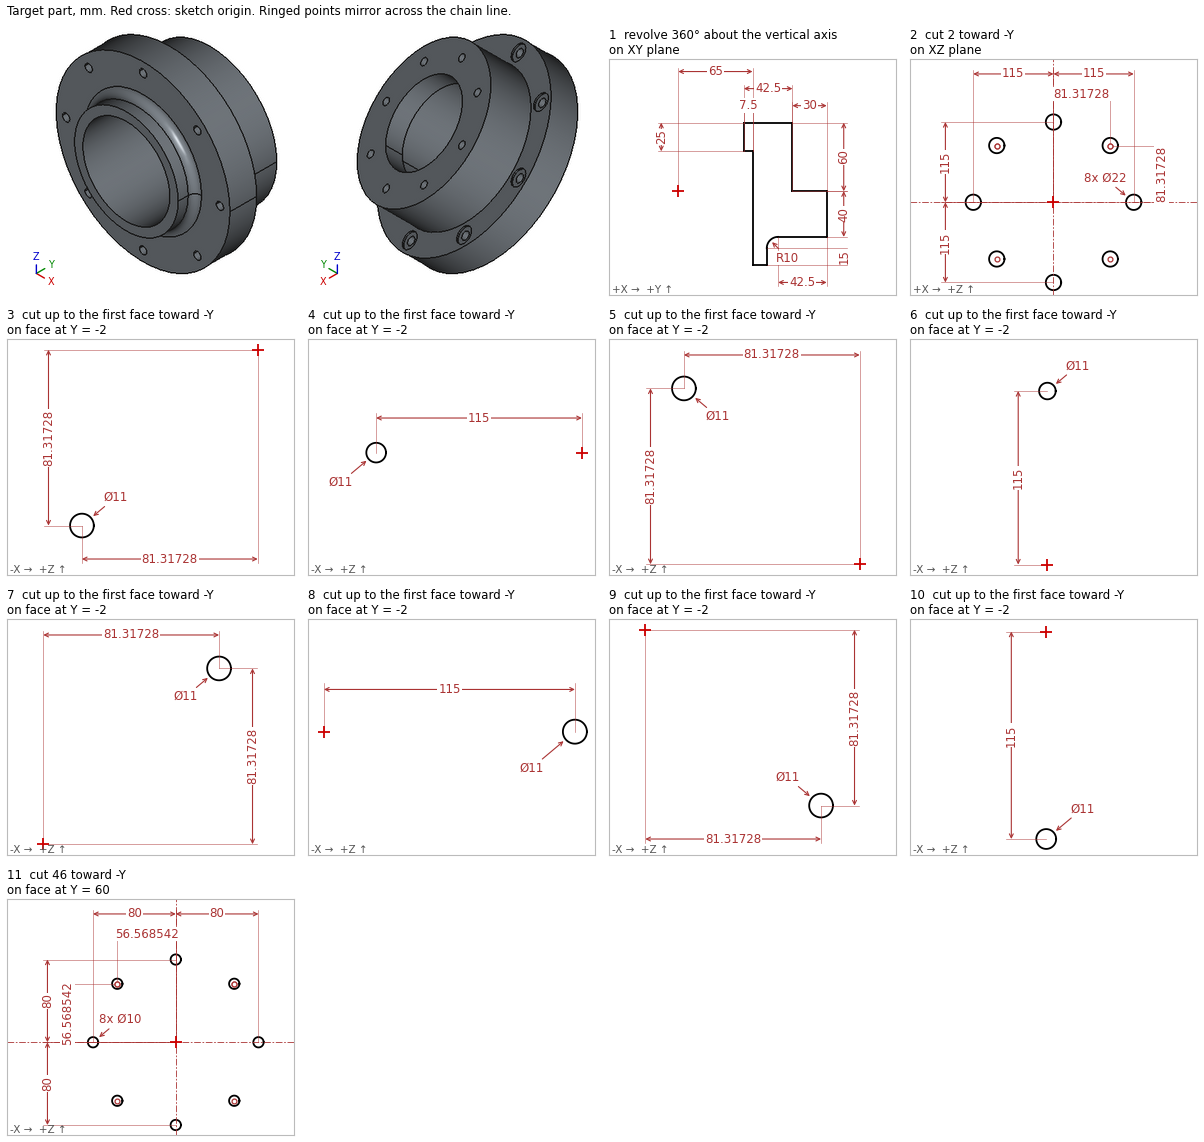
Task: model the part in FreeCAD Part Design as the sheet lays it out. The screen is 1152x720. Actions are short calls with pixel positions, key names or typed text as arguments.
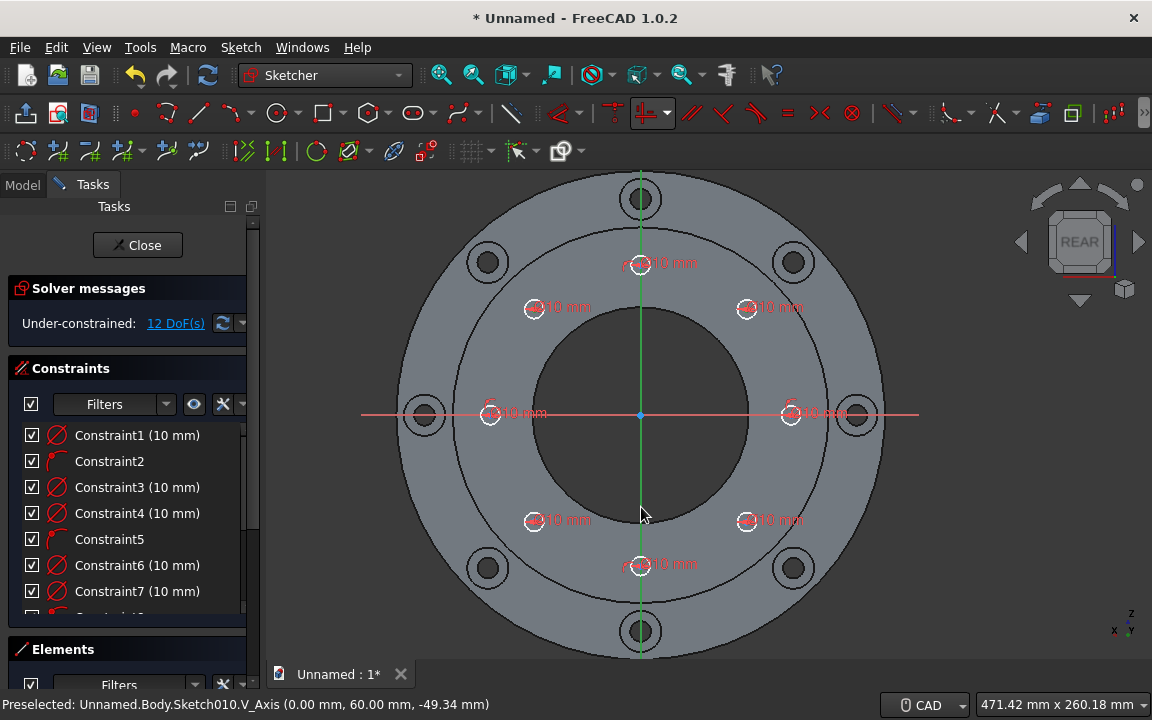
click(820, 114)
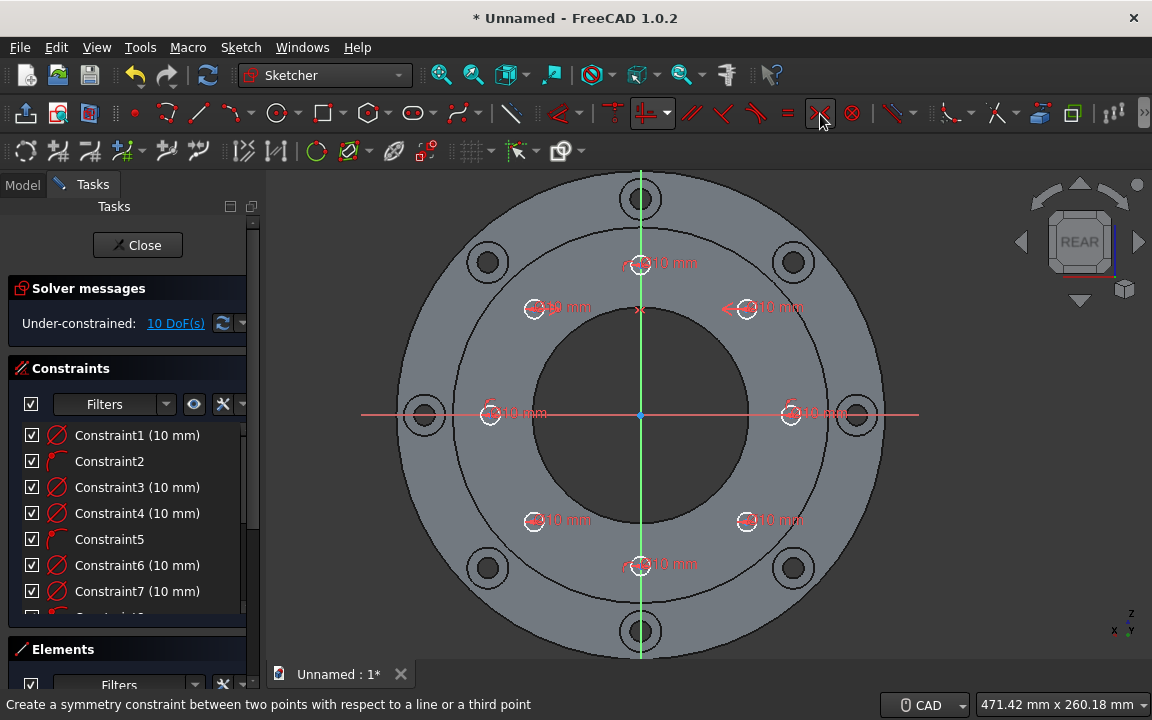
click(747, 309)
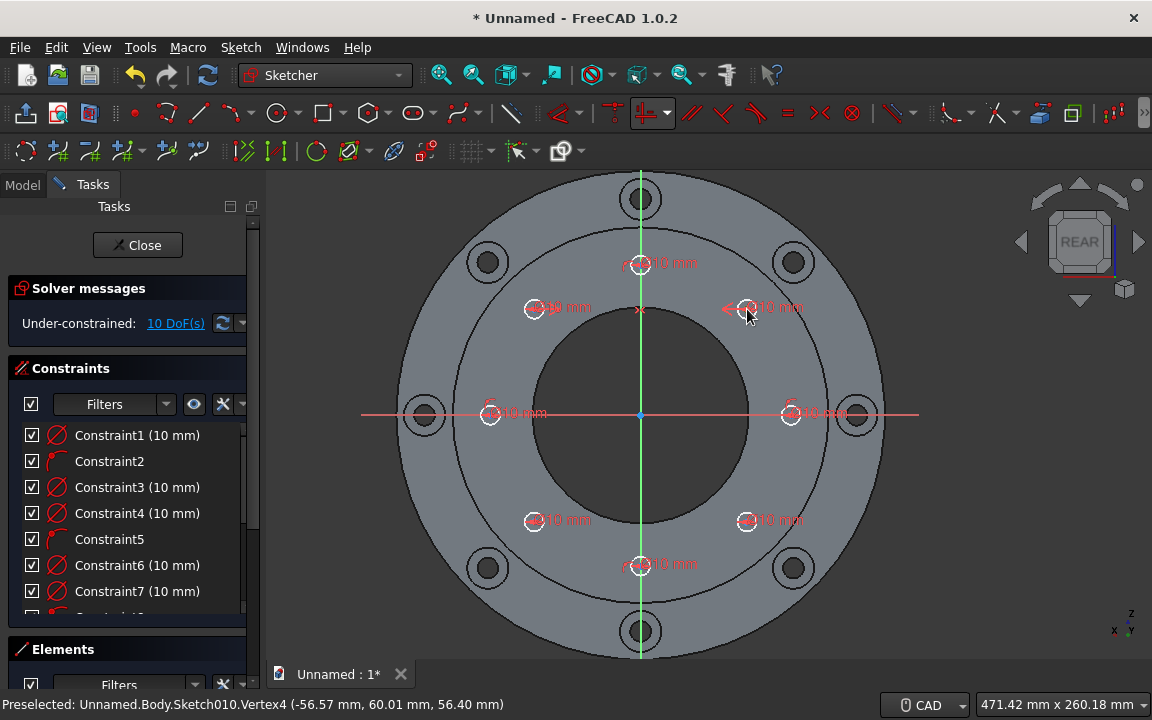
click(747, 522)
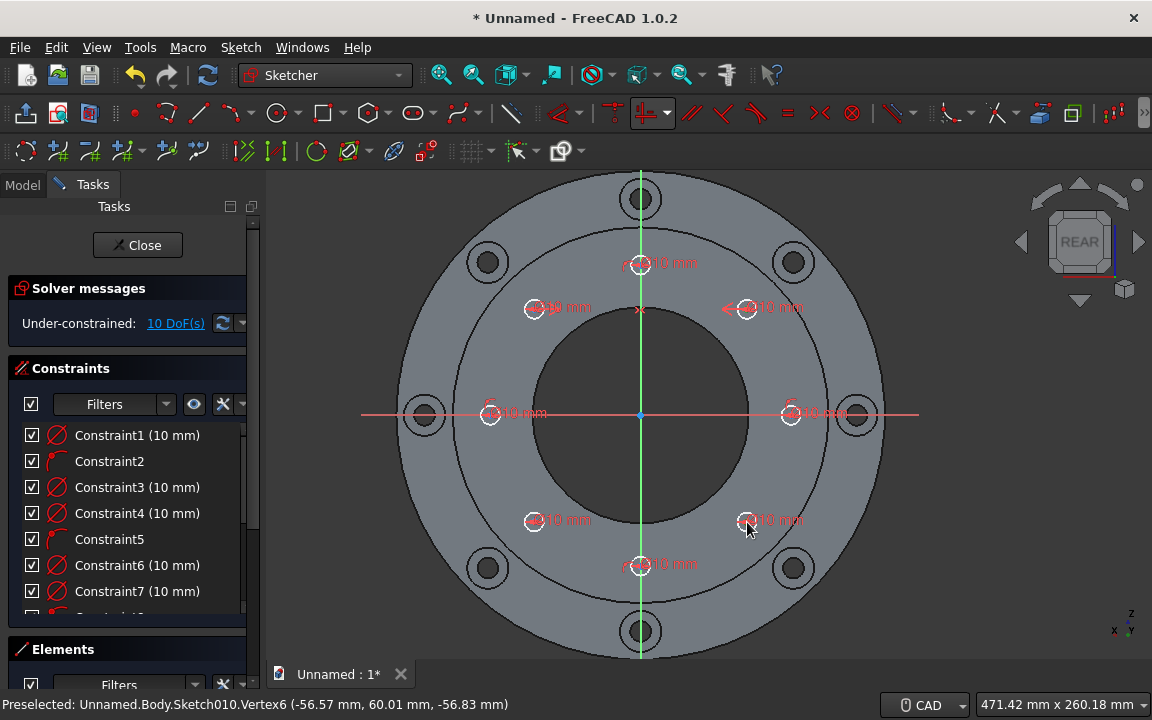
click(393, 415)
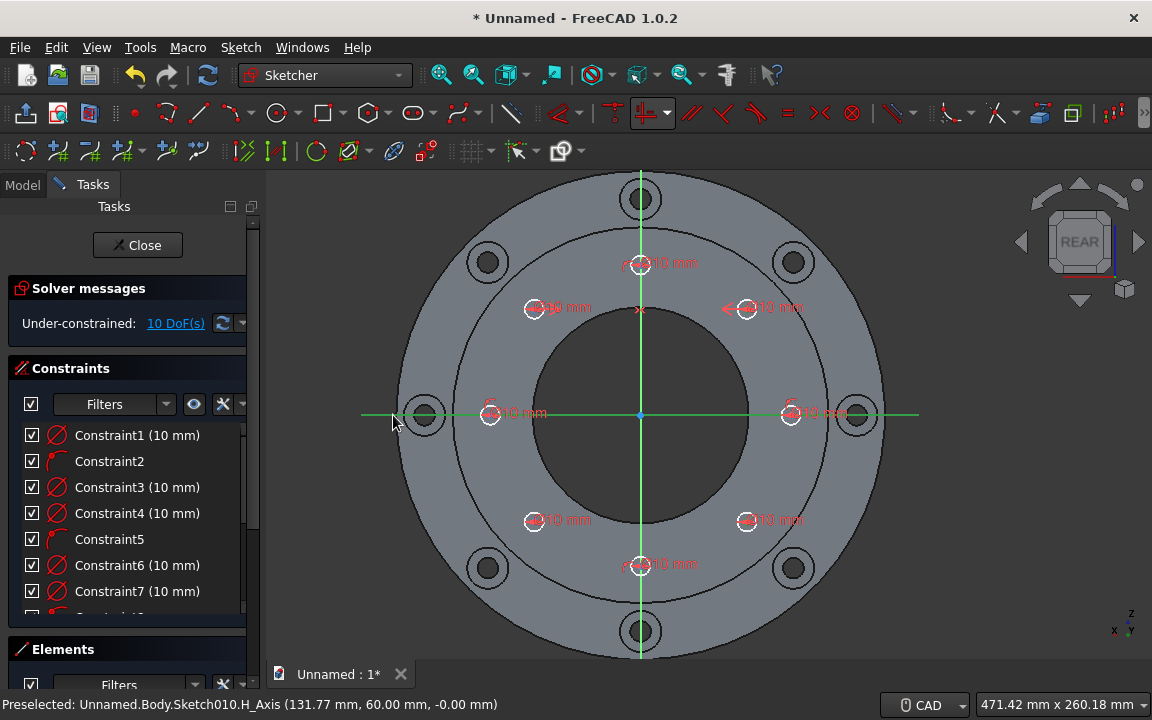
key(s)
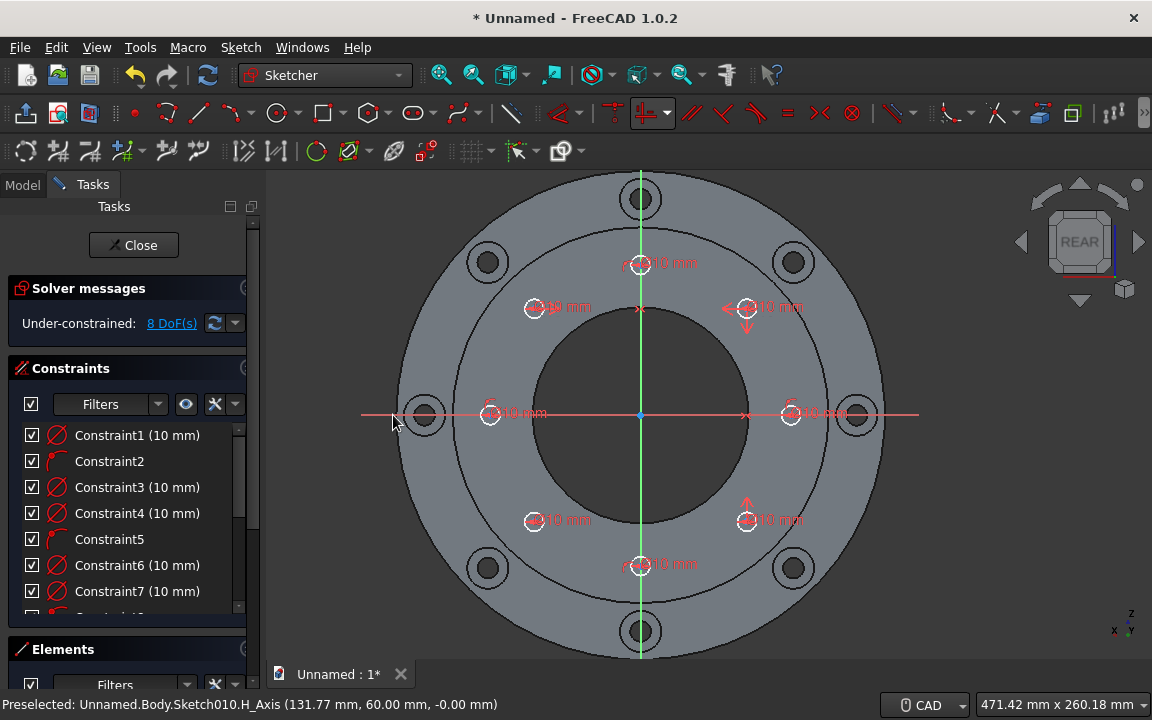
click(534, 309)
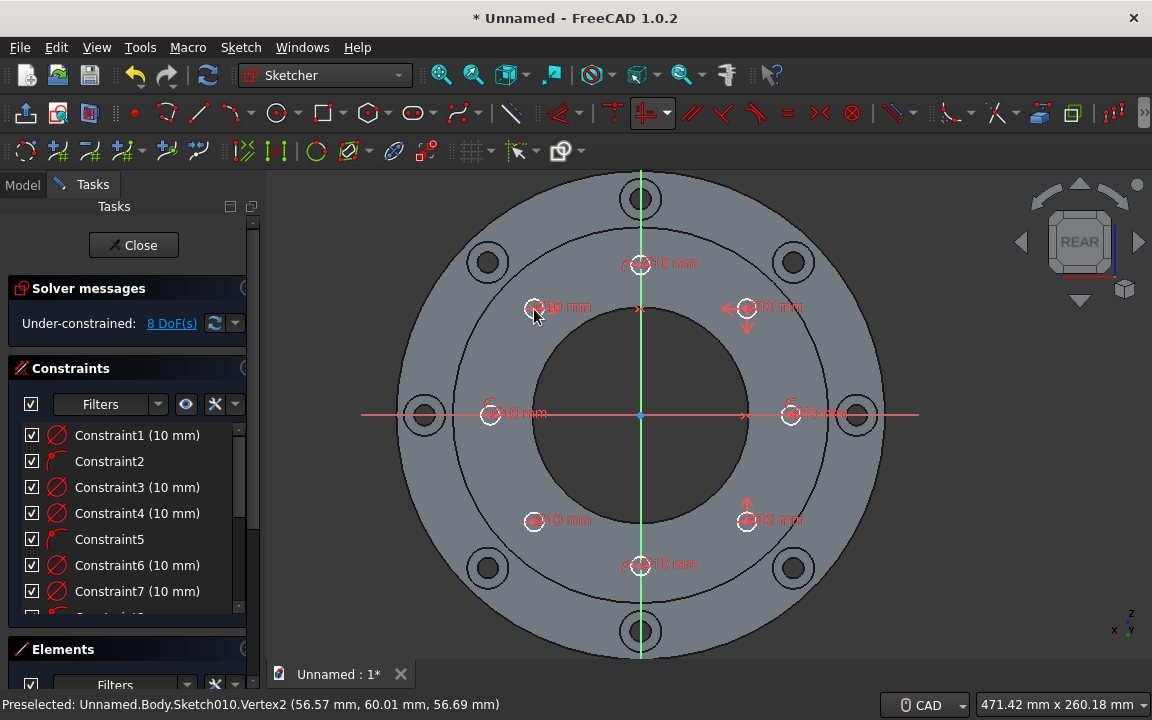
click(534, 522)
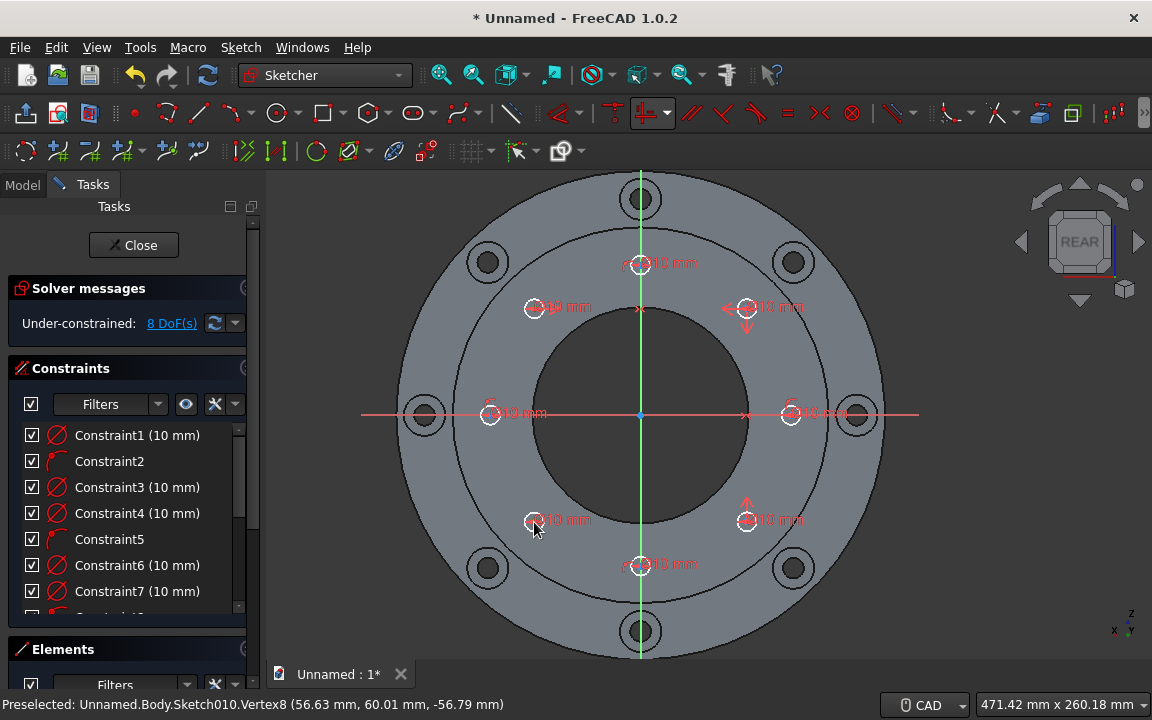
click(393, 415)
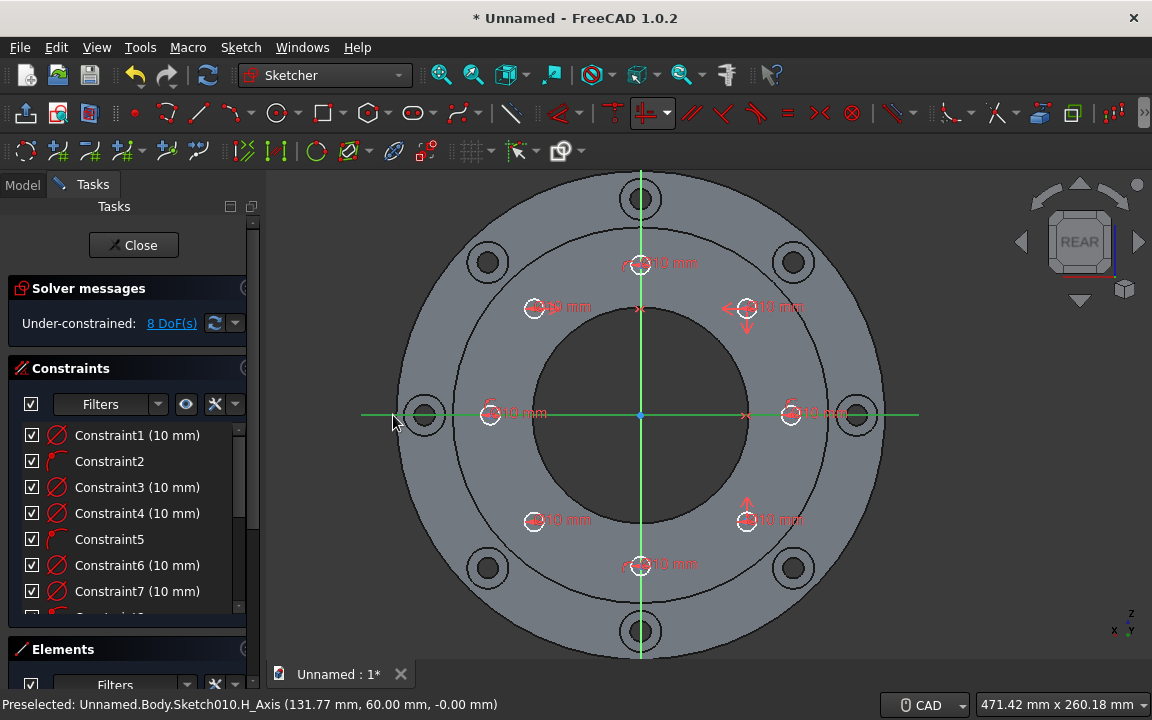
click(820, 114)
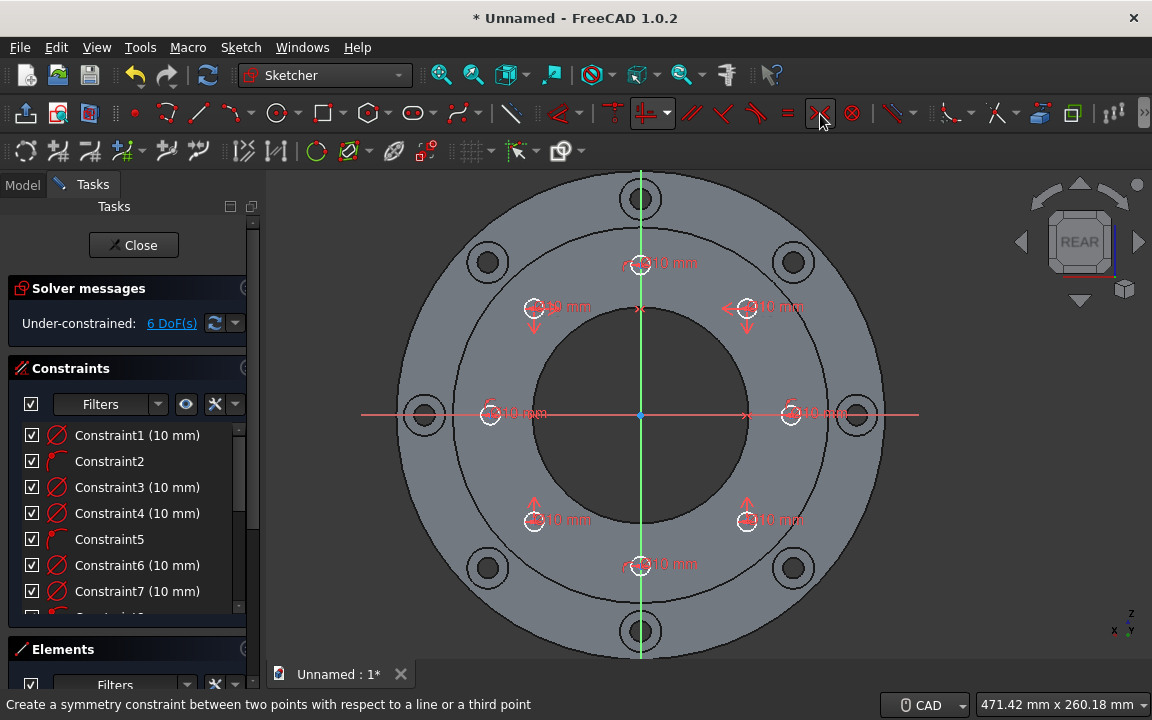
key(d)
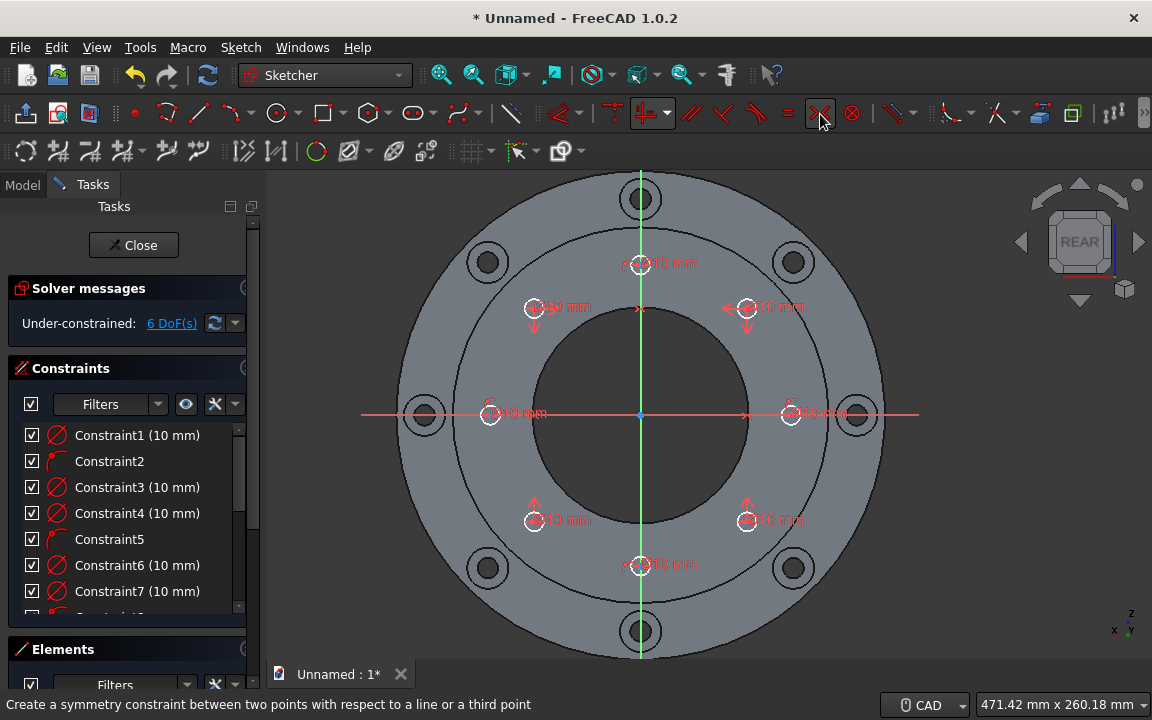
click(490, 415)
click(566, 449)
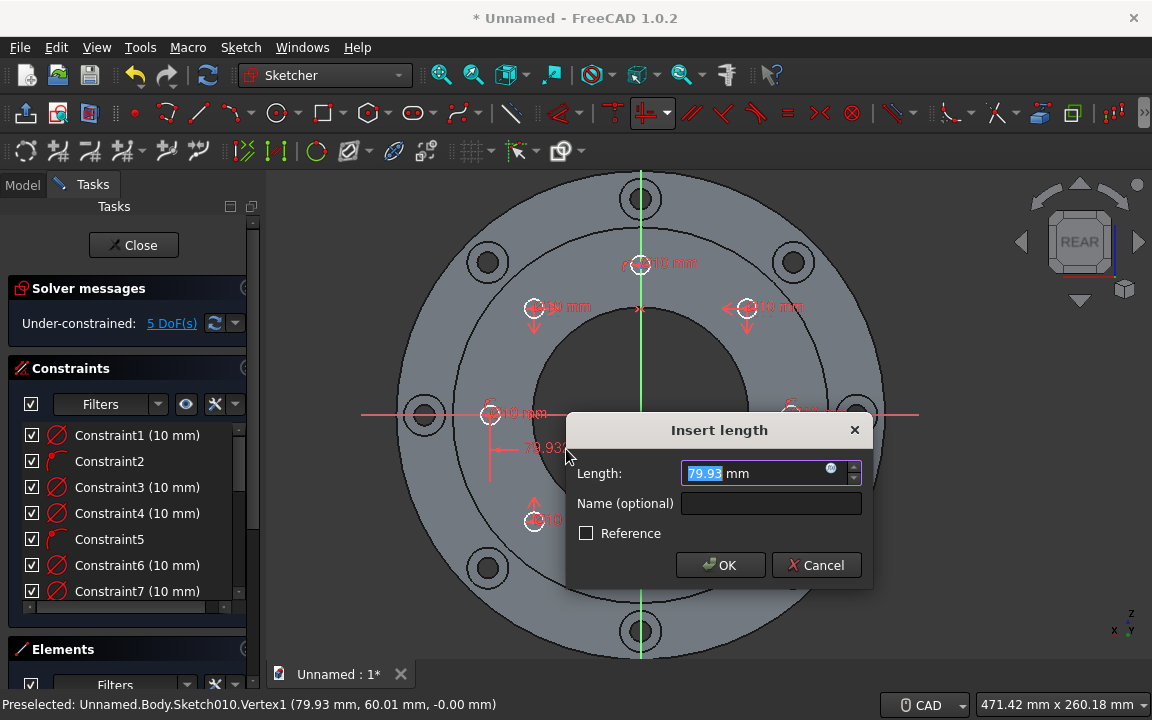
text(80)
key(Return)